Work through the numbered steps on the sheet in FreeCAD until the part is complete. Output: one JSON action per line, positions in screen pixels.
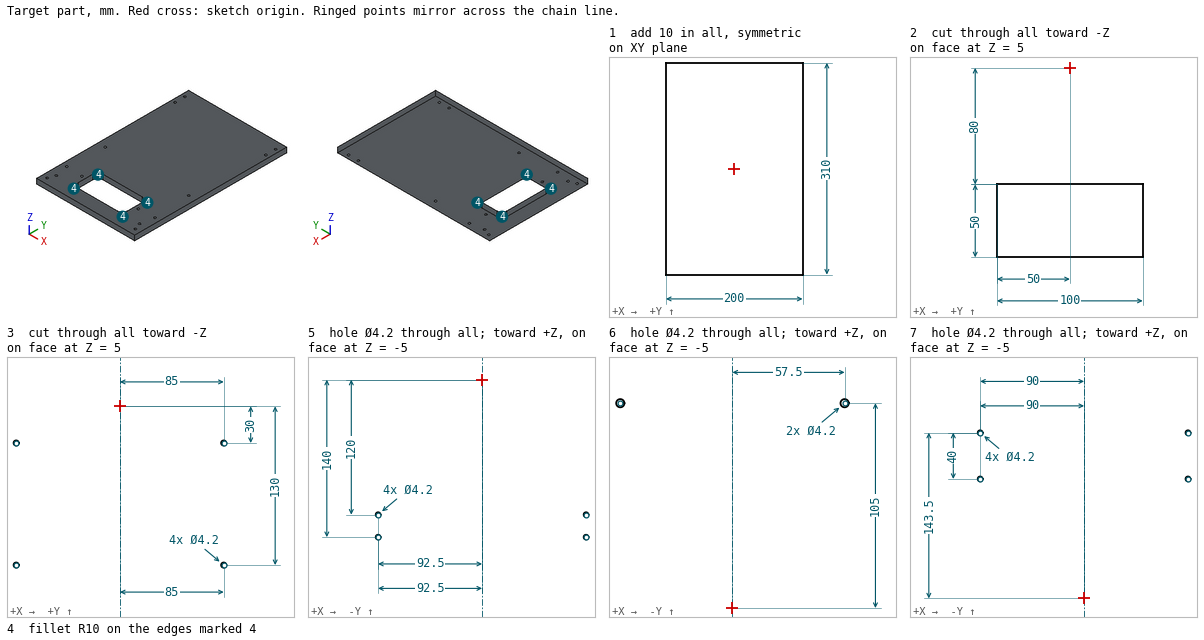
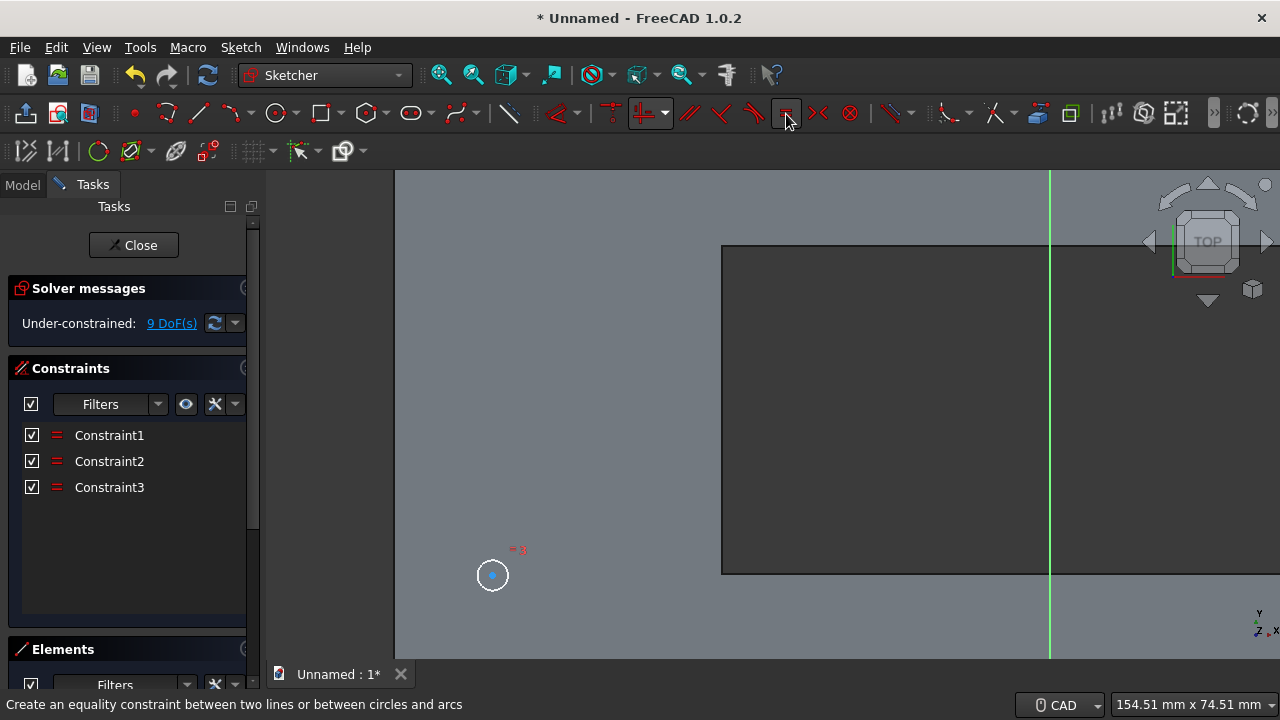
{"action": "scroll", "coordinate": [503, 566], "scroll_direction": "down", "scroll_amount": 5}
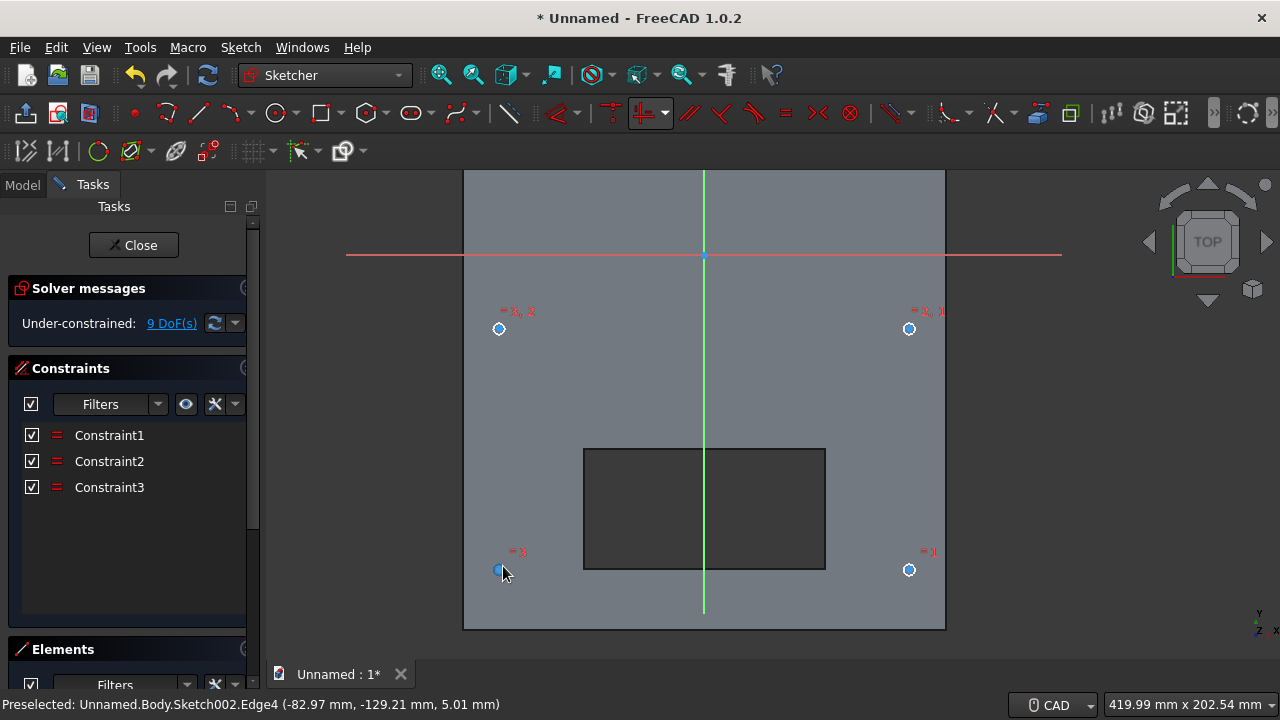
{"action": "left_click", "coordinate": [909, 329]}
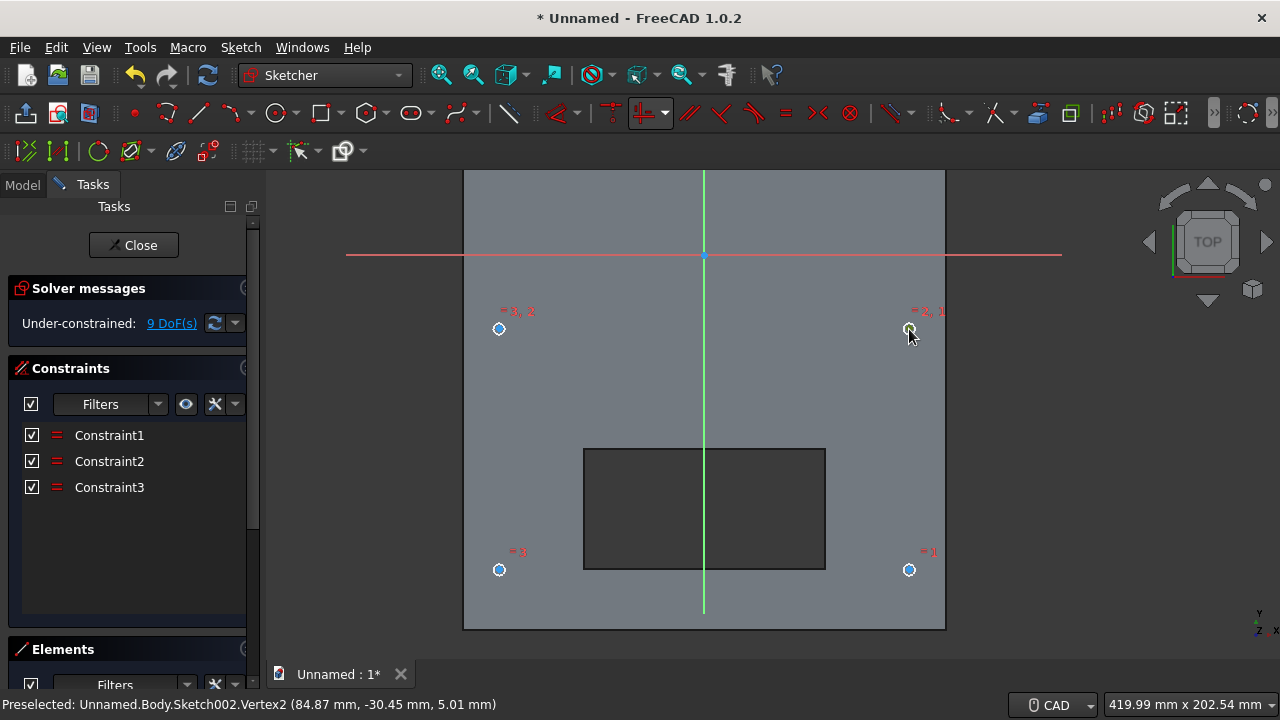
{"action": "left_click", "coordinate": [499, 329]}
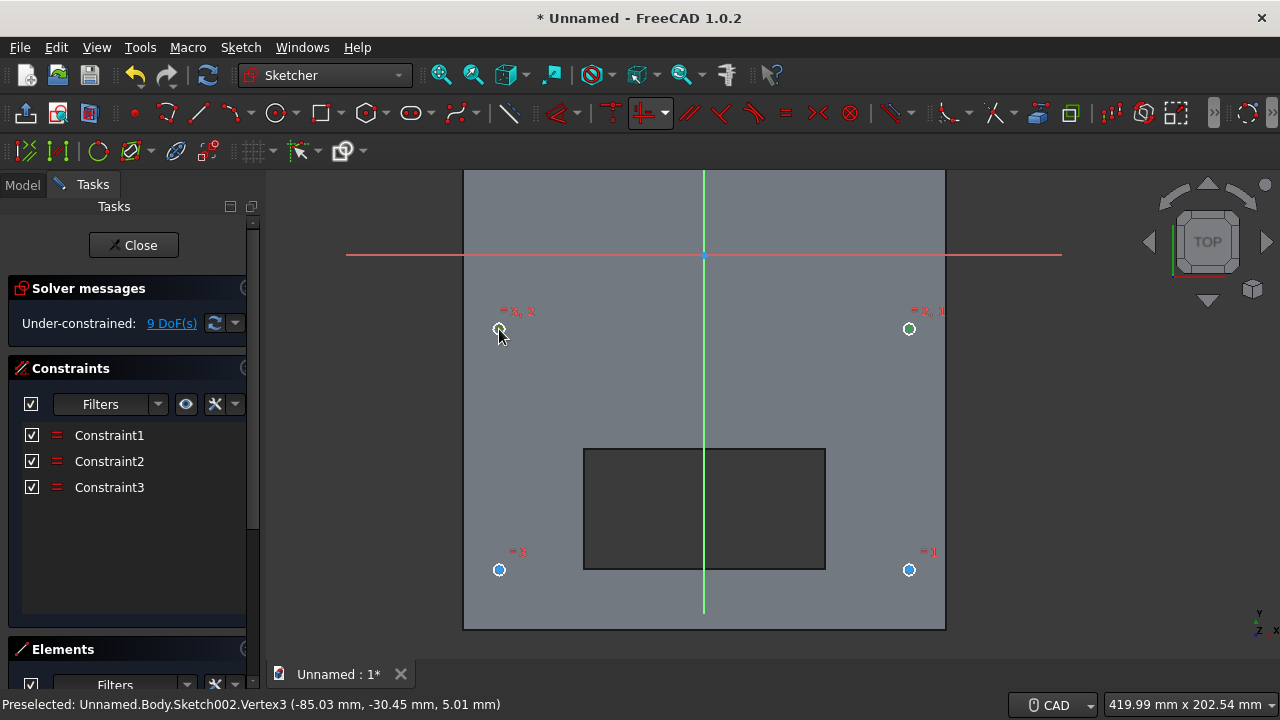
{"action": "left_click", "coordinate": [704, 600]}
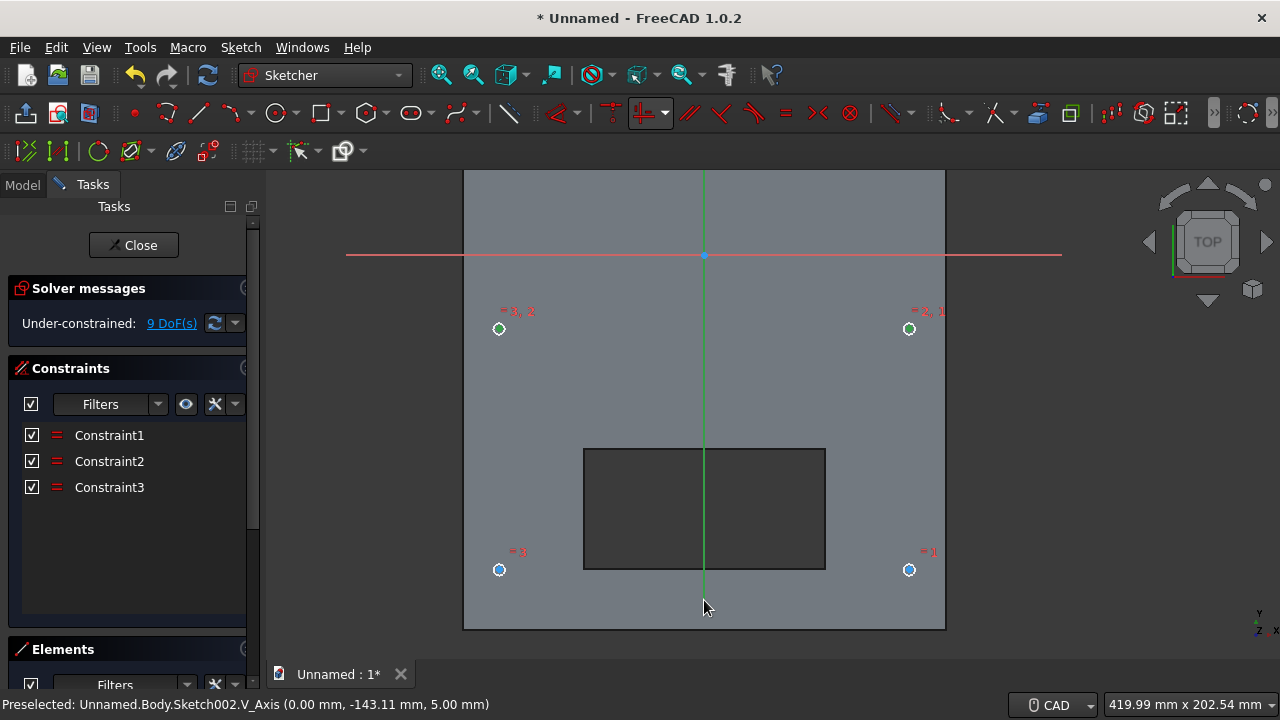
{"action": "left_click", "coordinate": [818, 114]}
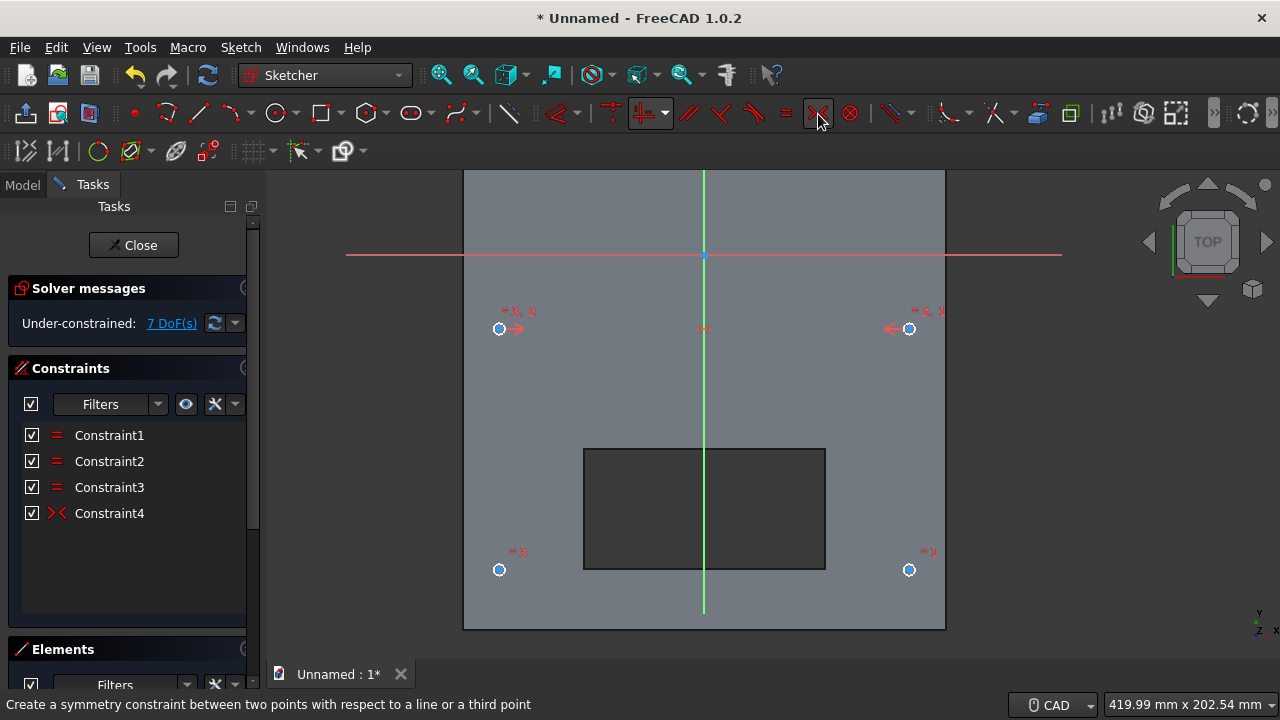
{"action": "left_click", "coordinate": [909, 570]}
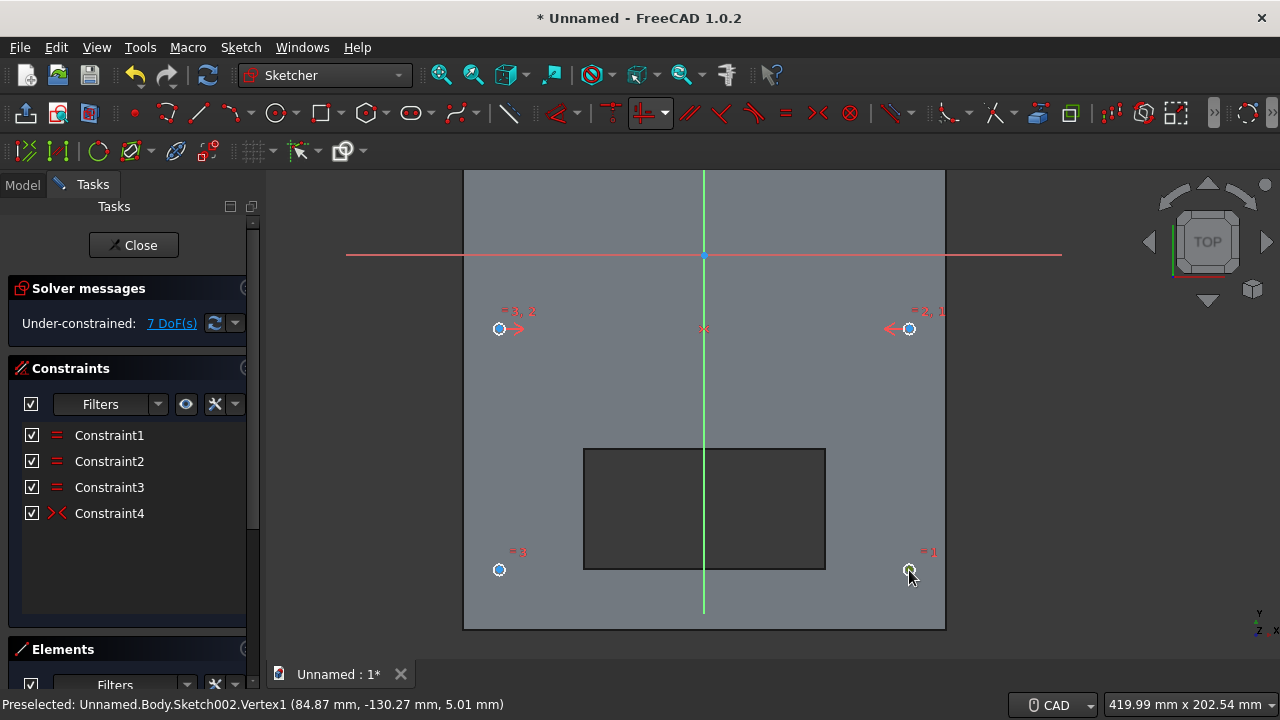
{"action": "left_click", "coordinate": [499, 570]}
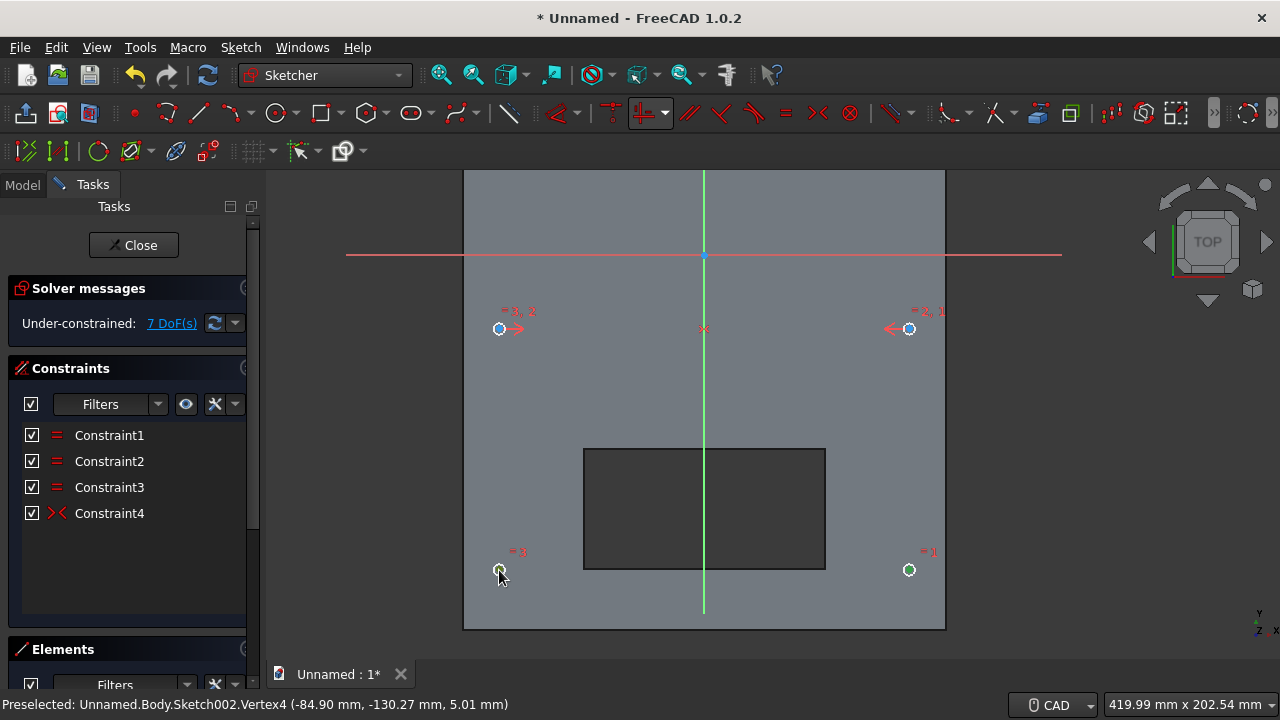
{"action": "left_click", "coordinate": [704, 600]}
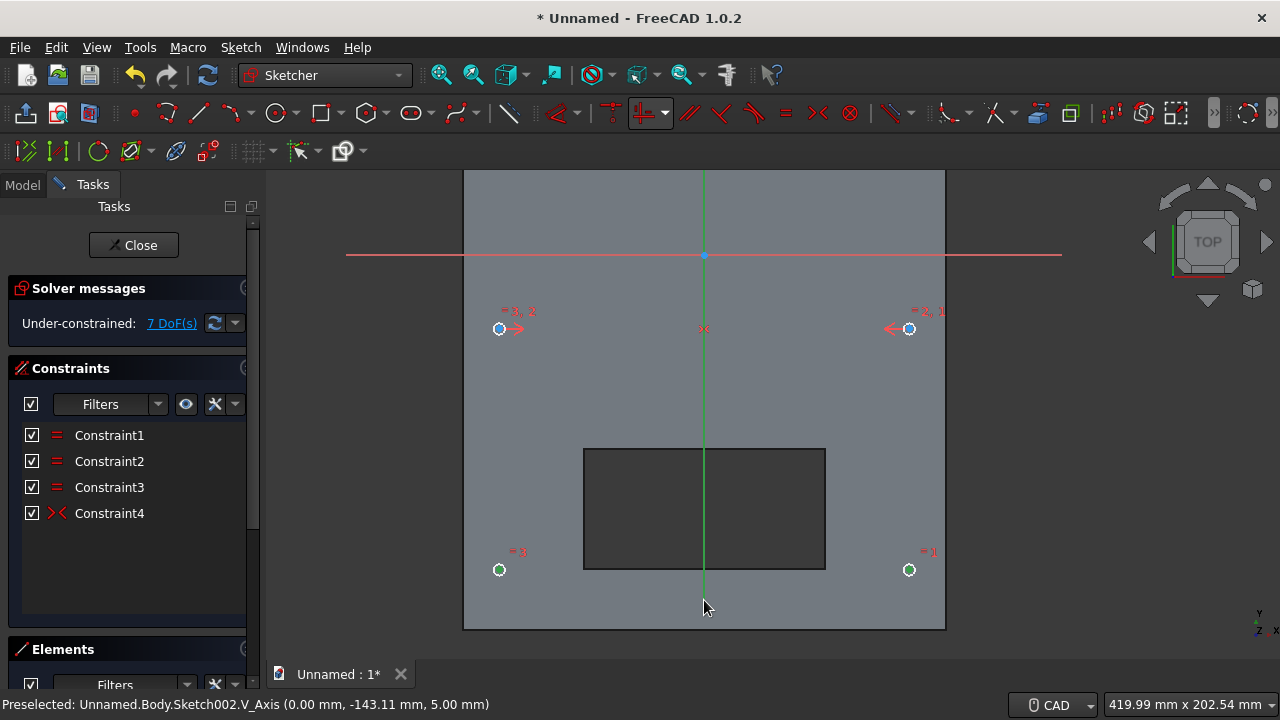
{"action": "left_click", "coordinate": [818, 114]}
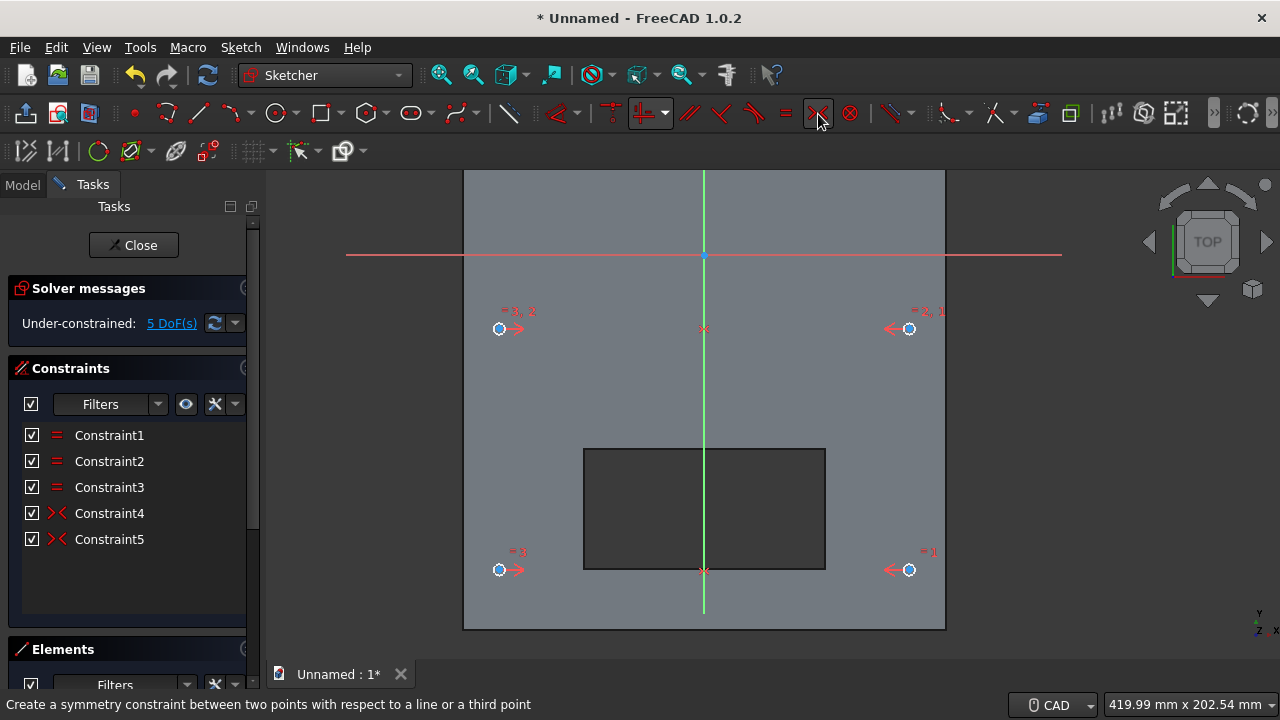
{"action": "left_click", "coordinate": [556, 114]}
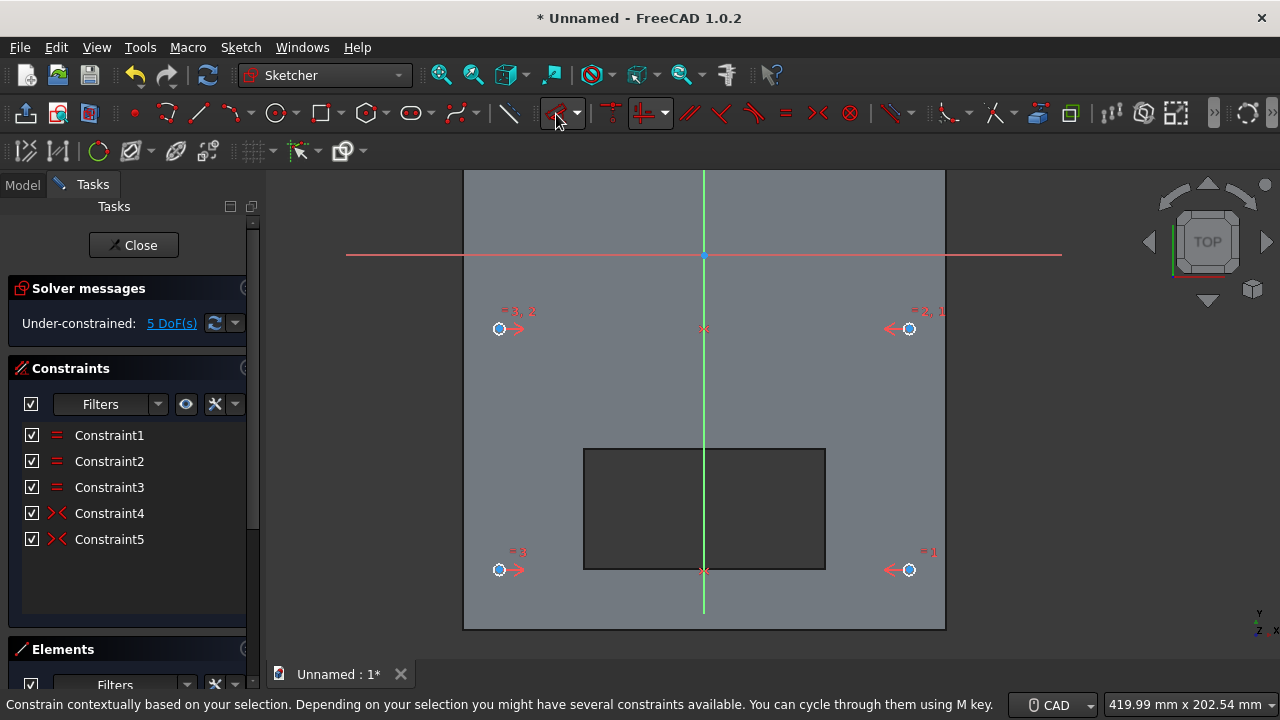
{"action": "scroll", "coordinate": [913, 566], "scroll_direction": "up", "scroll_amount": 7}